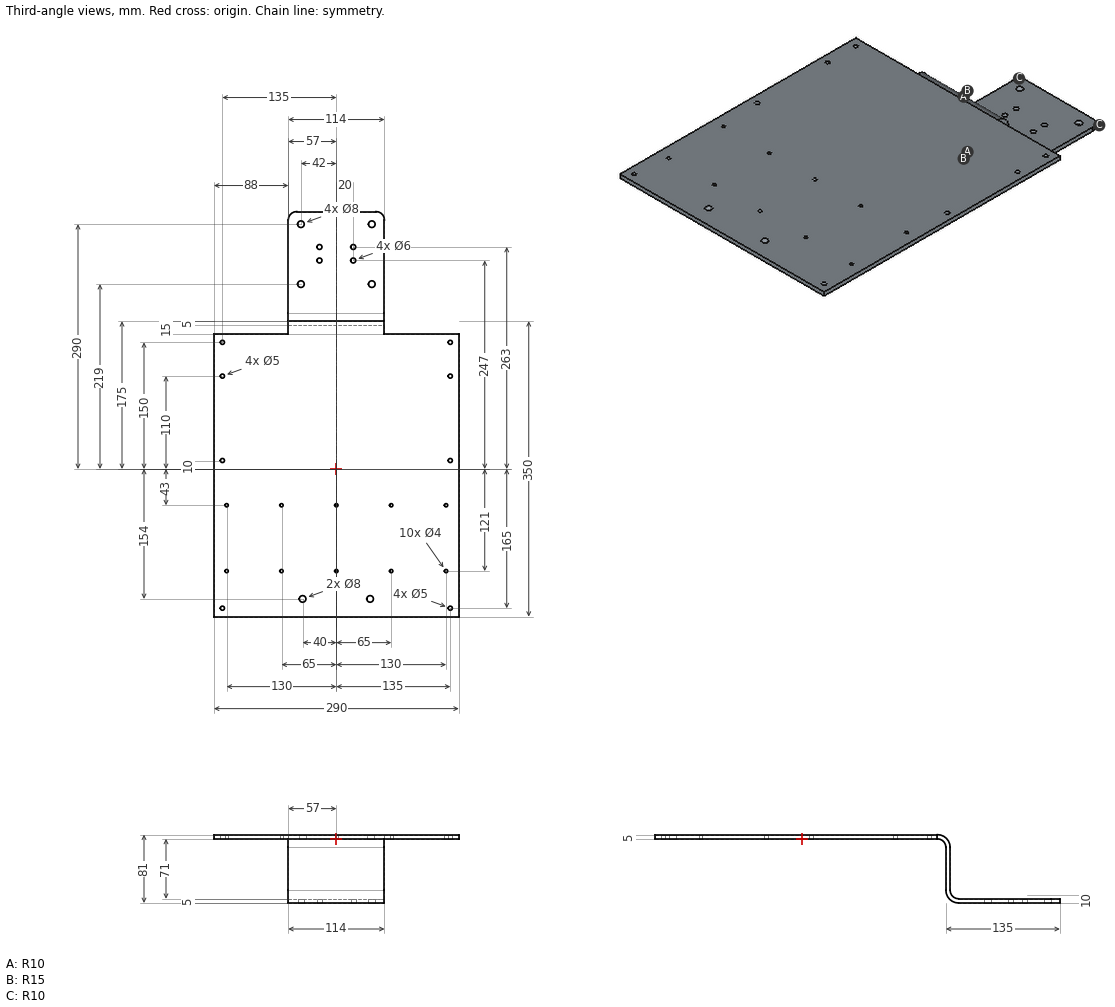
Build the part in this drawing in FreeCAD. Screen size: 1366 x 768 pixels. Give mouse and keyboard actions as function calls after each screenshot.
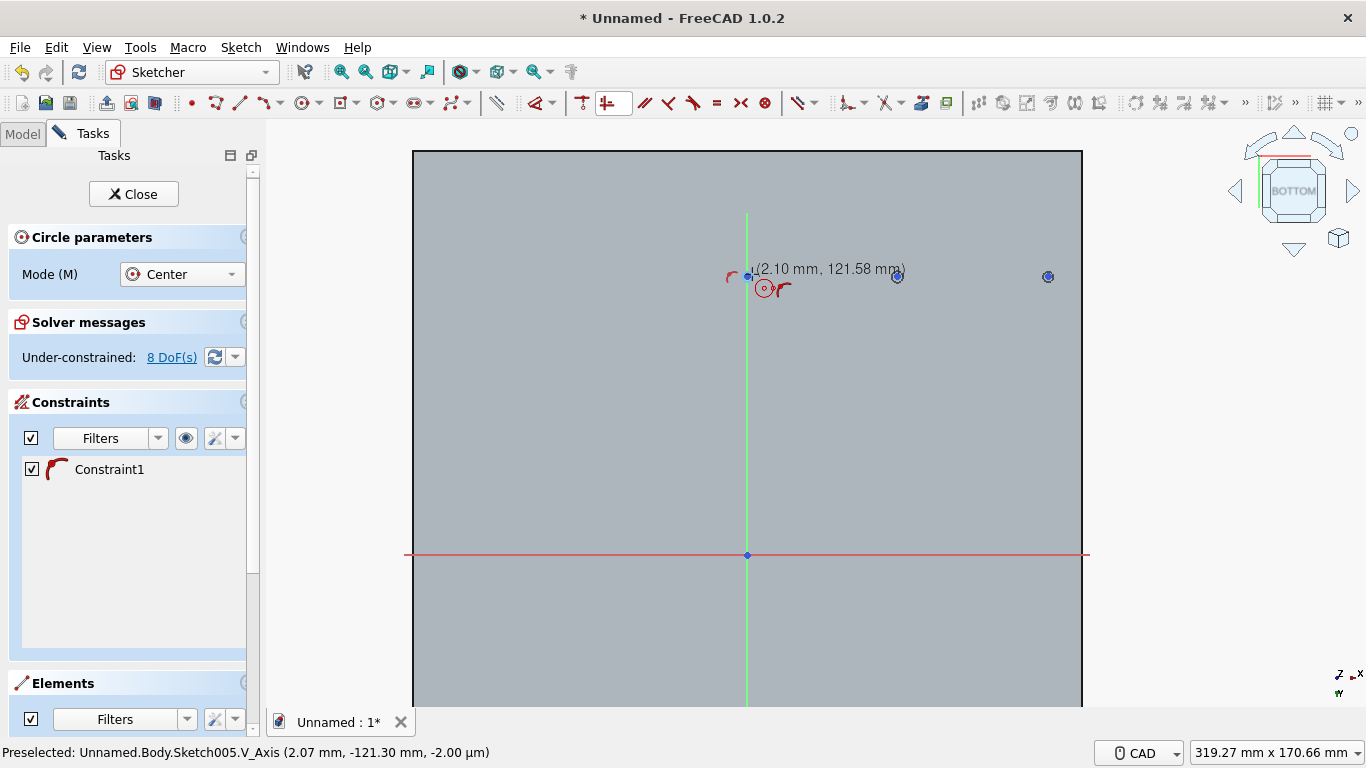
scroll(597, 276, up, 8)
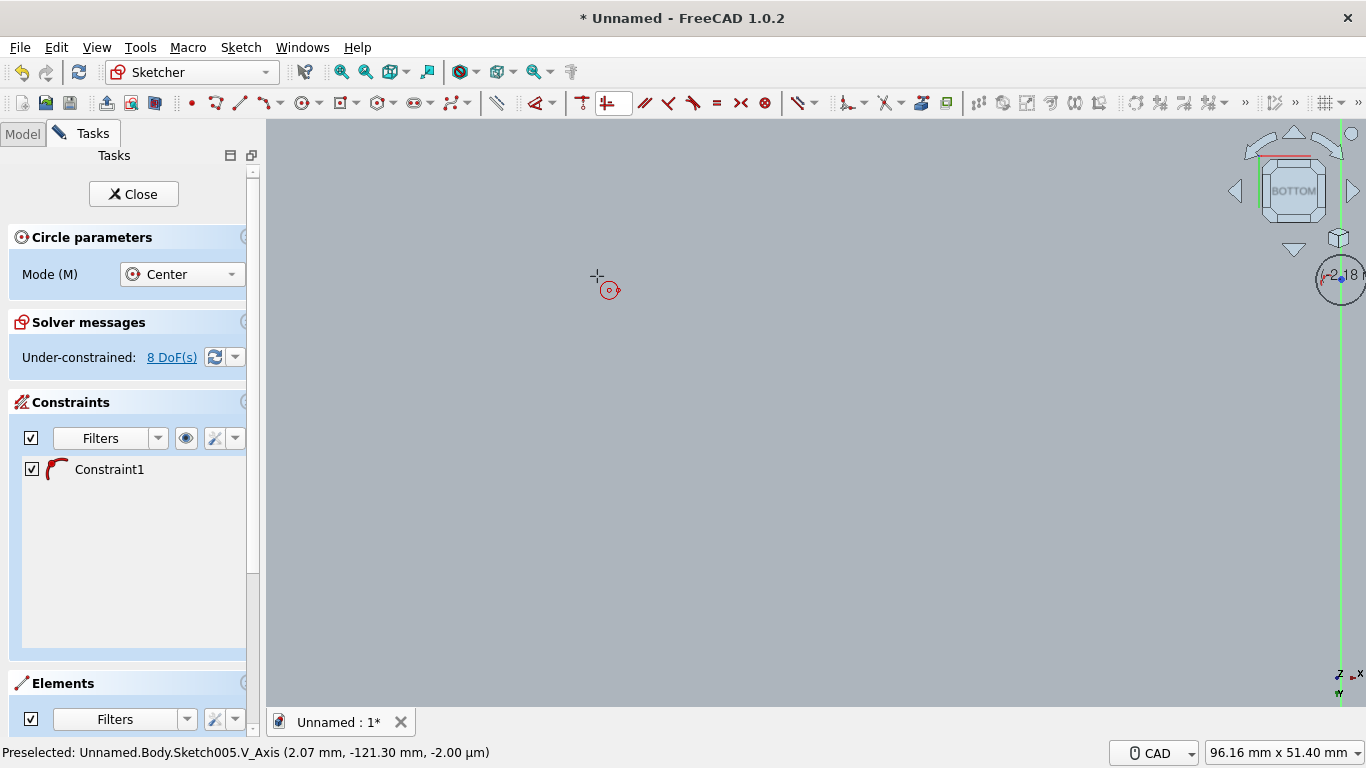
scroll(597, 276, down, 8)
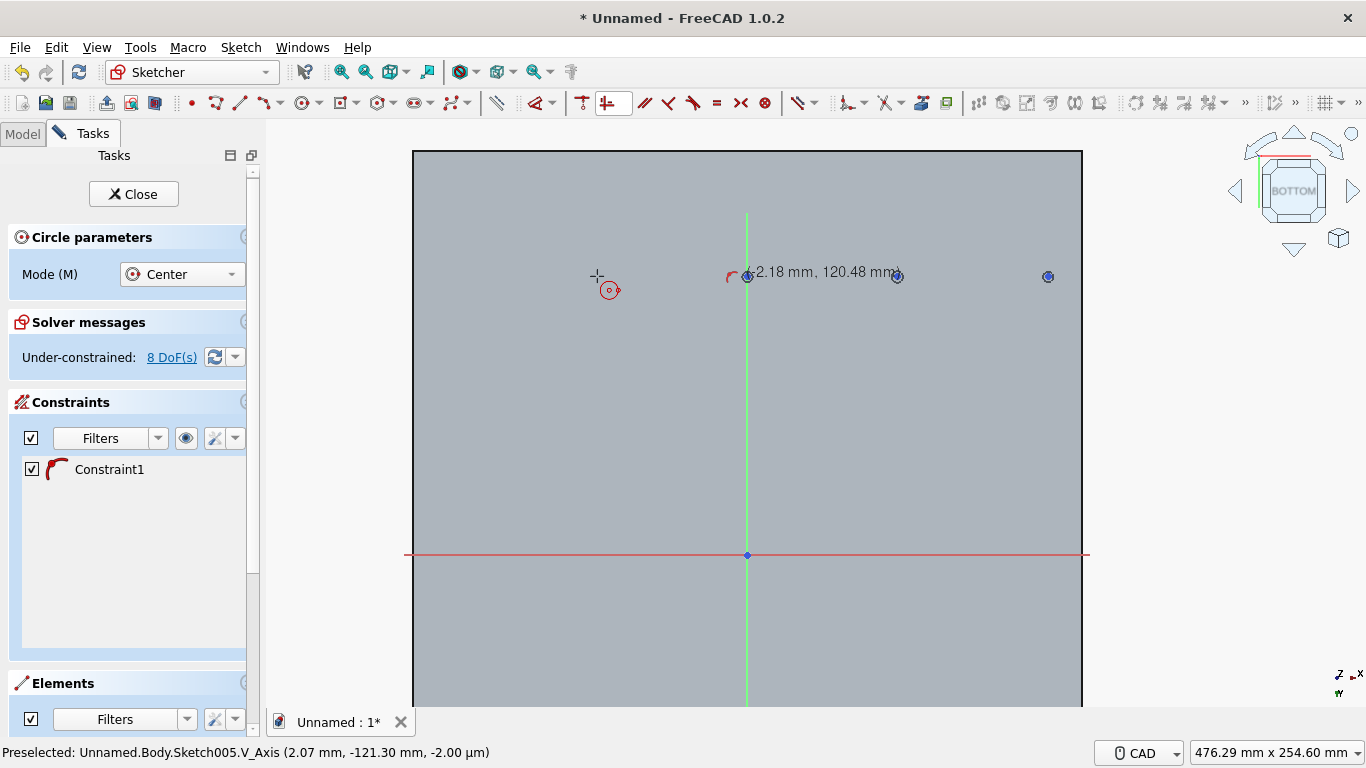
click(597, 276)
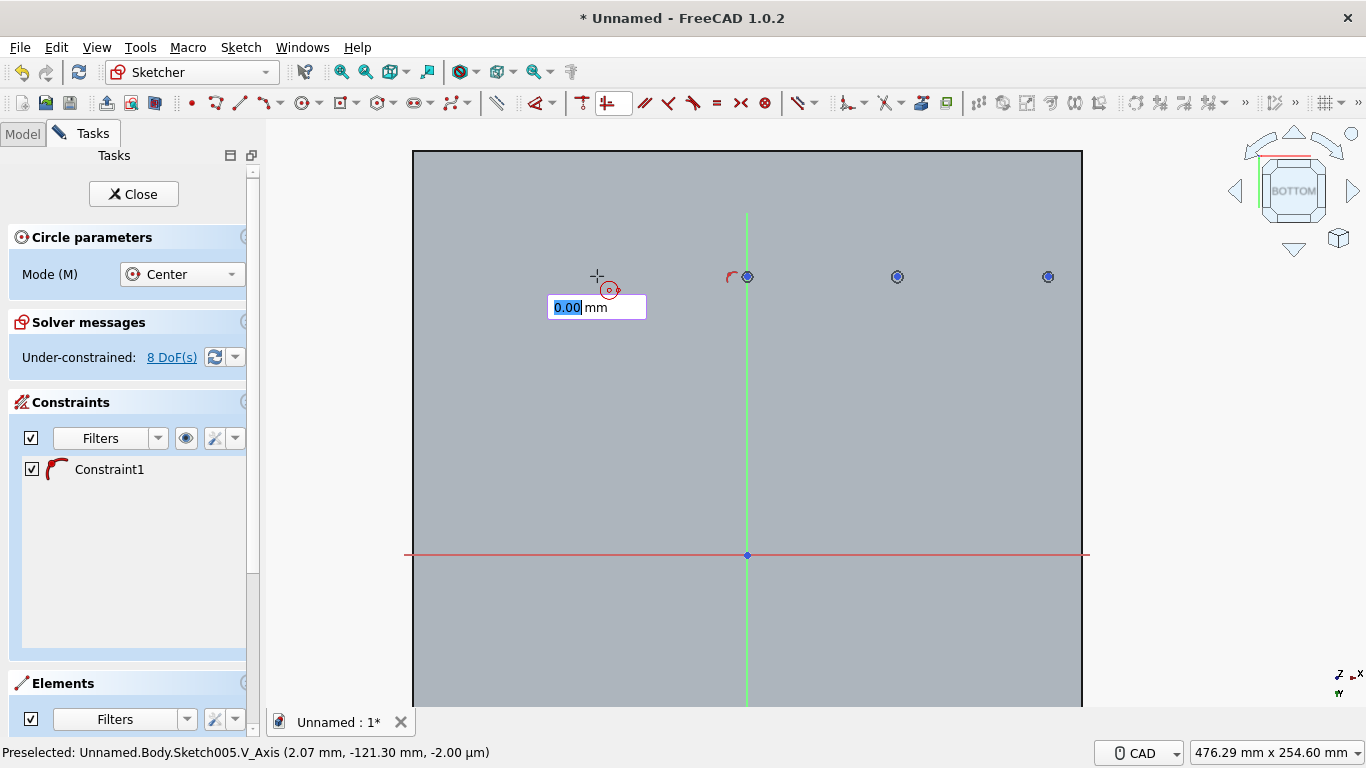
scroll(601, 273, up, 7)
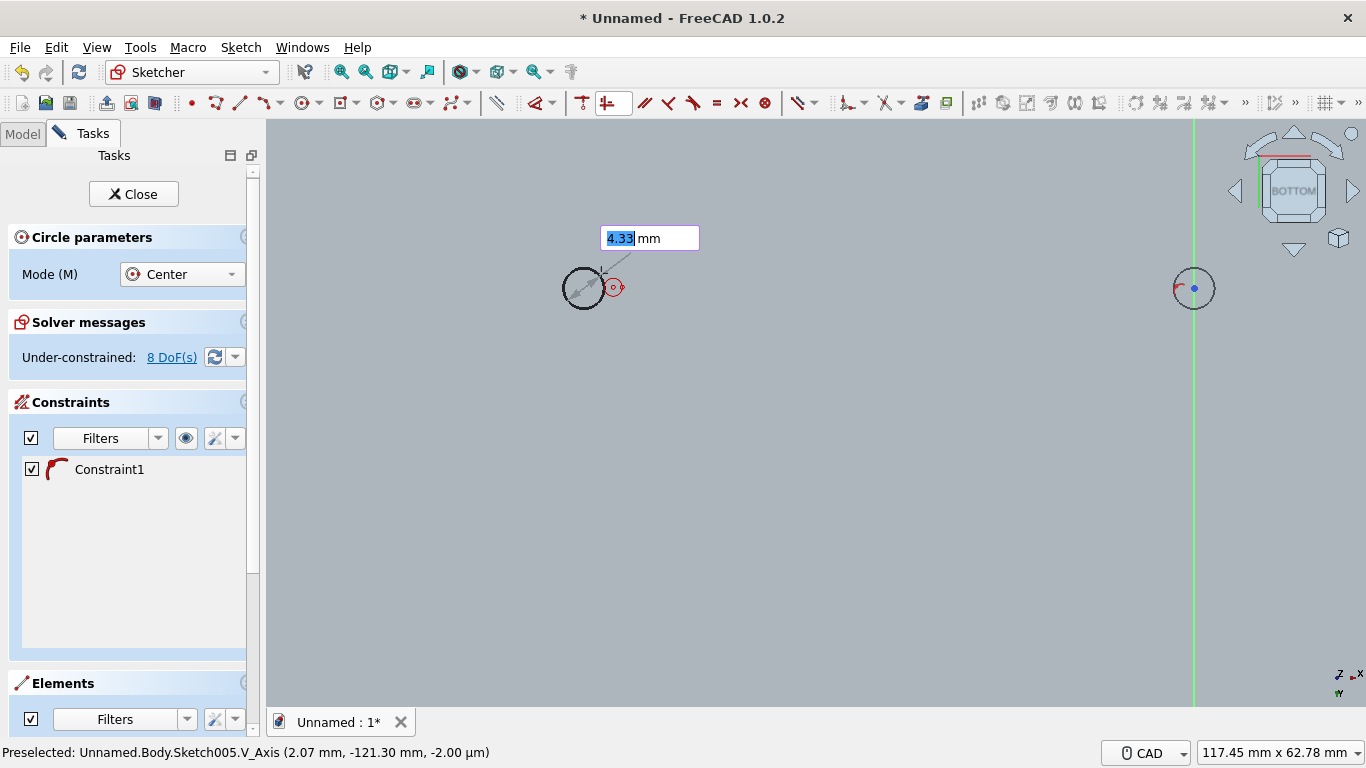
click(599, 270)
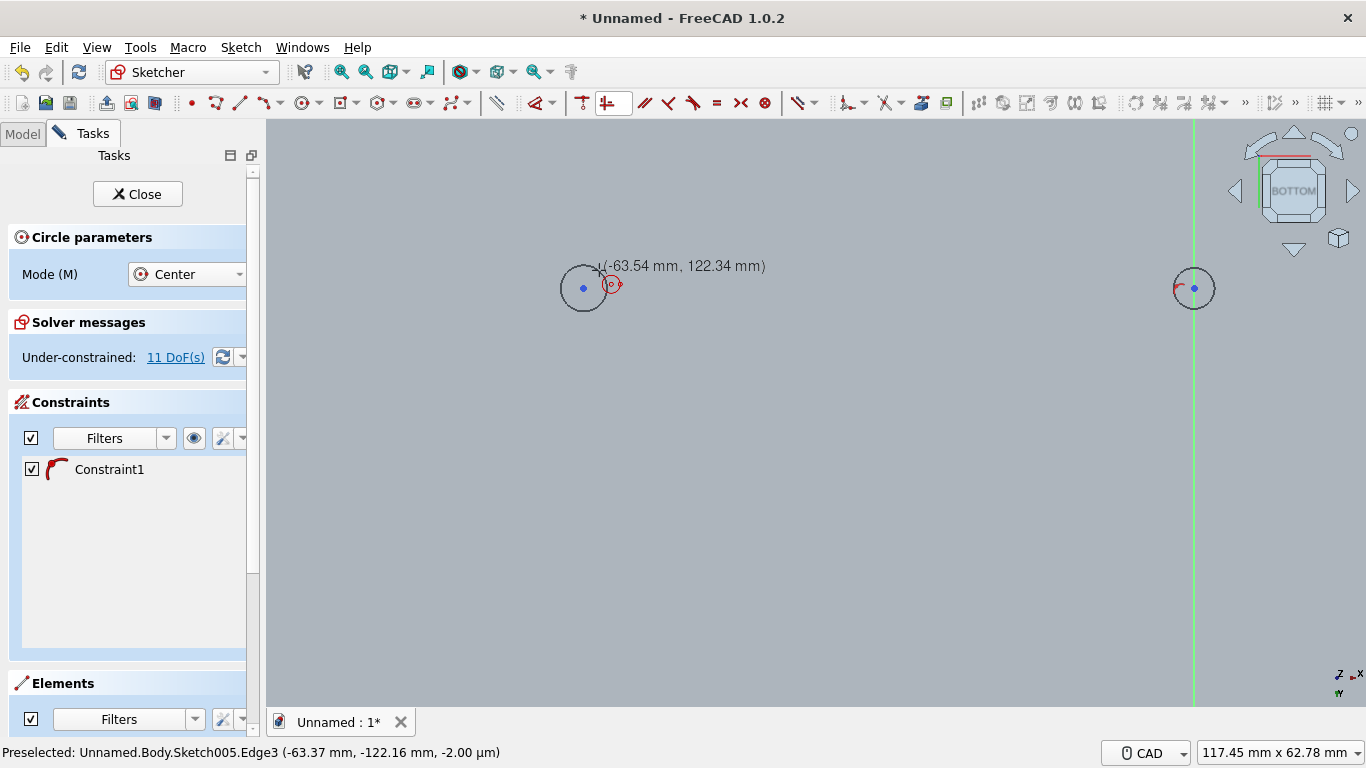
scroll(601, 273, down, 7)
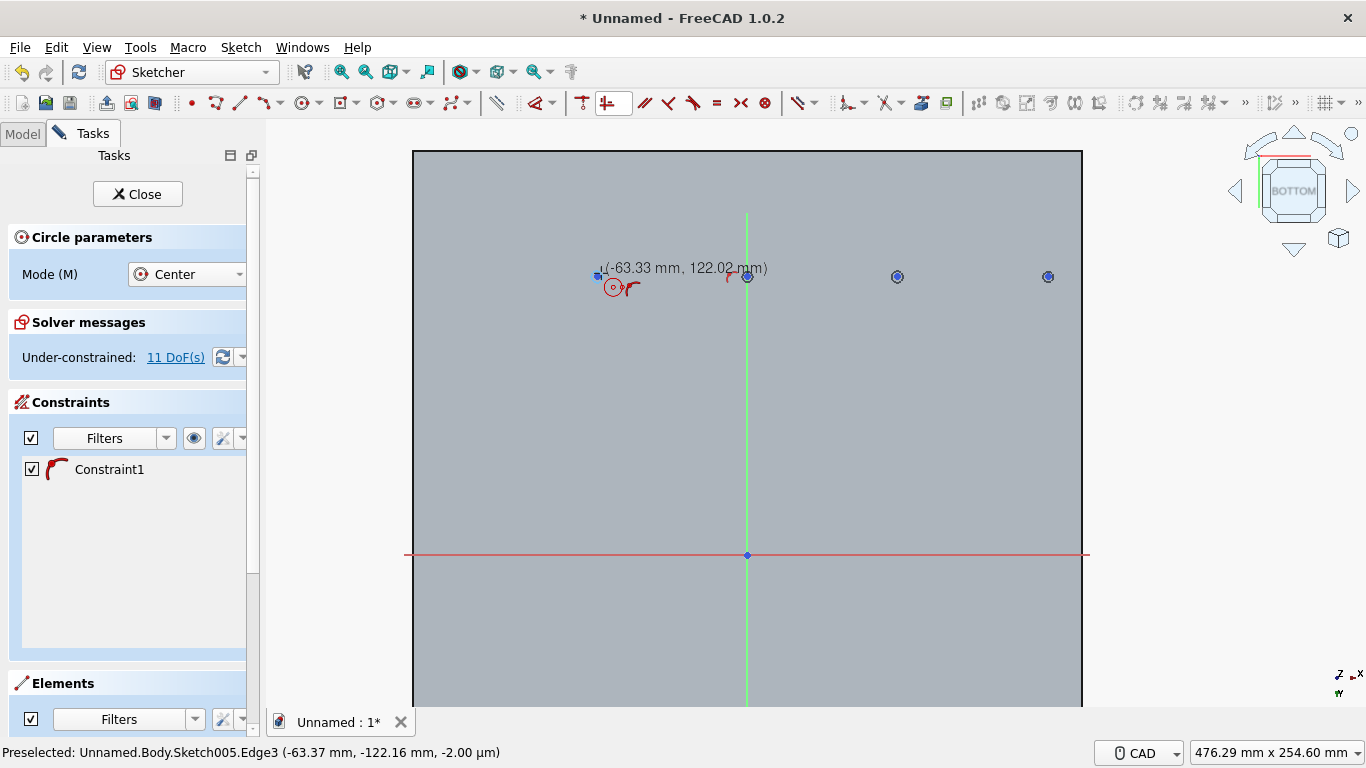
scroll(447, 276, up, 8)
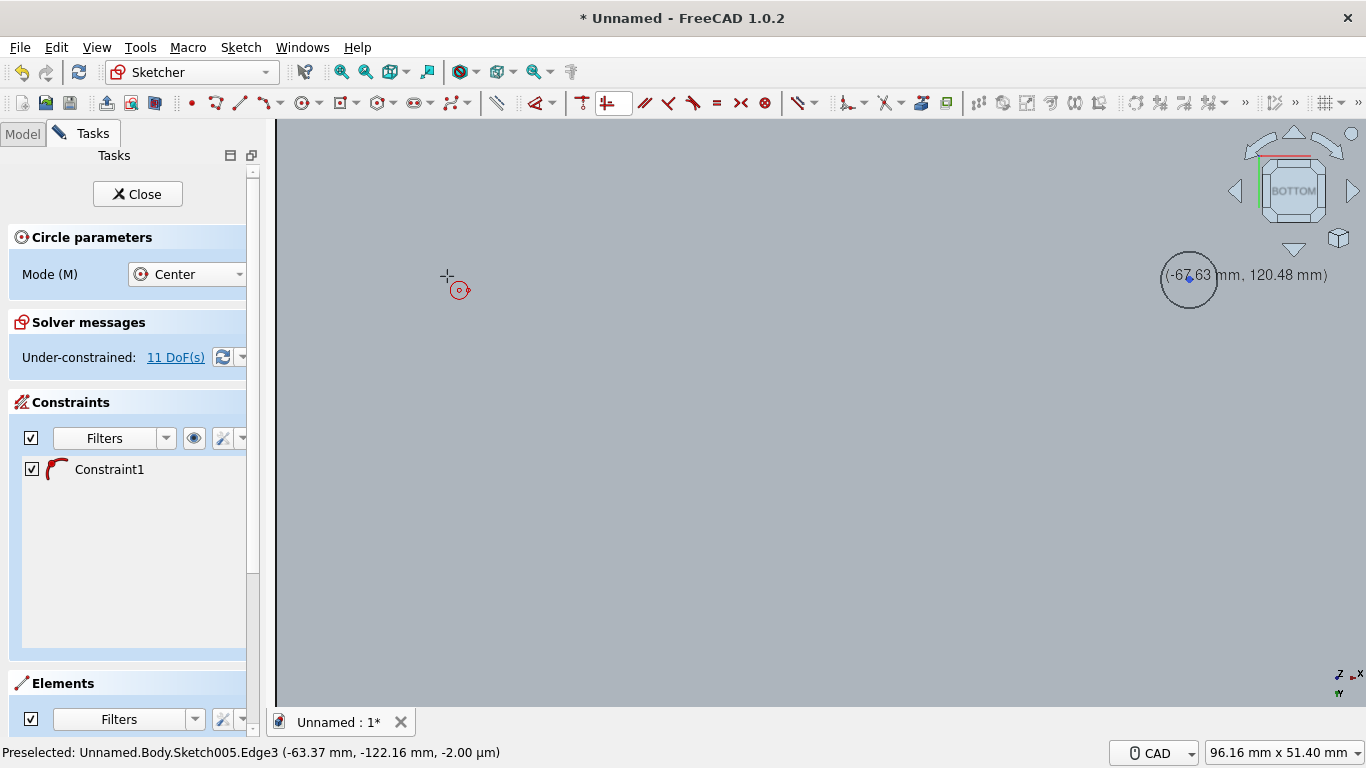
scroll(447, 276, down, 8)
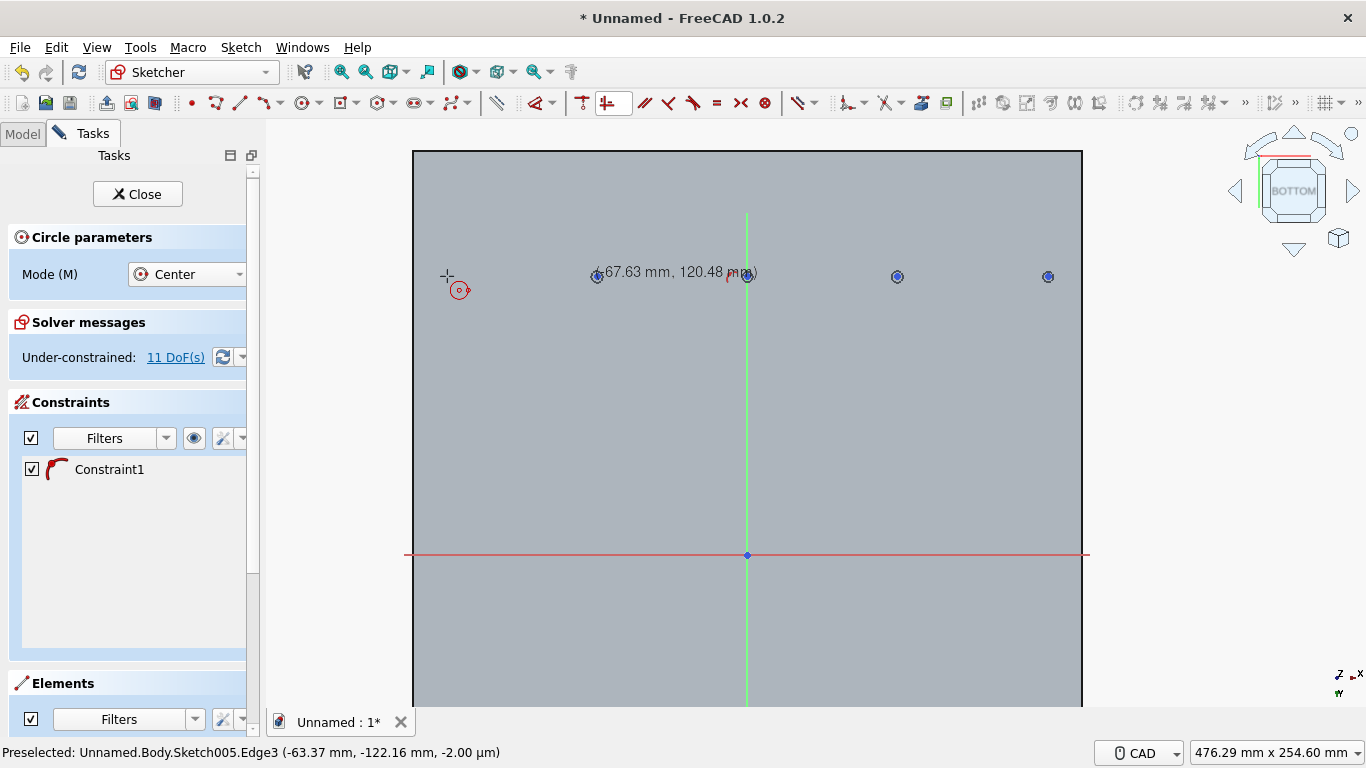
click(447, 276)